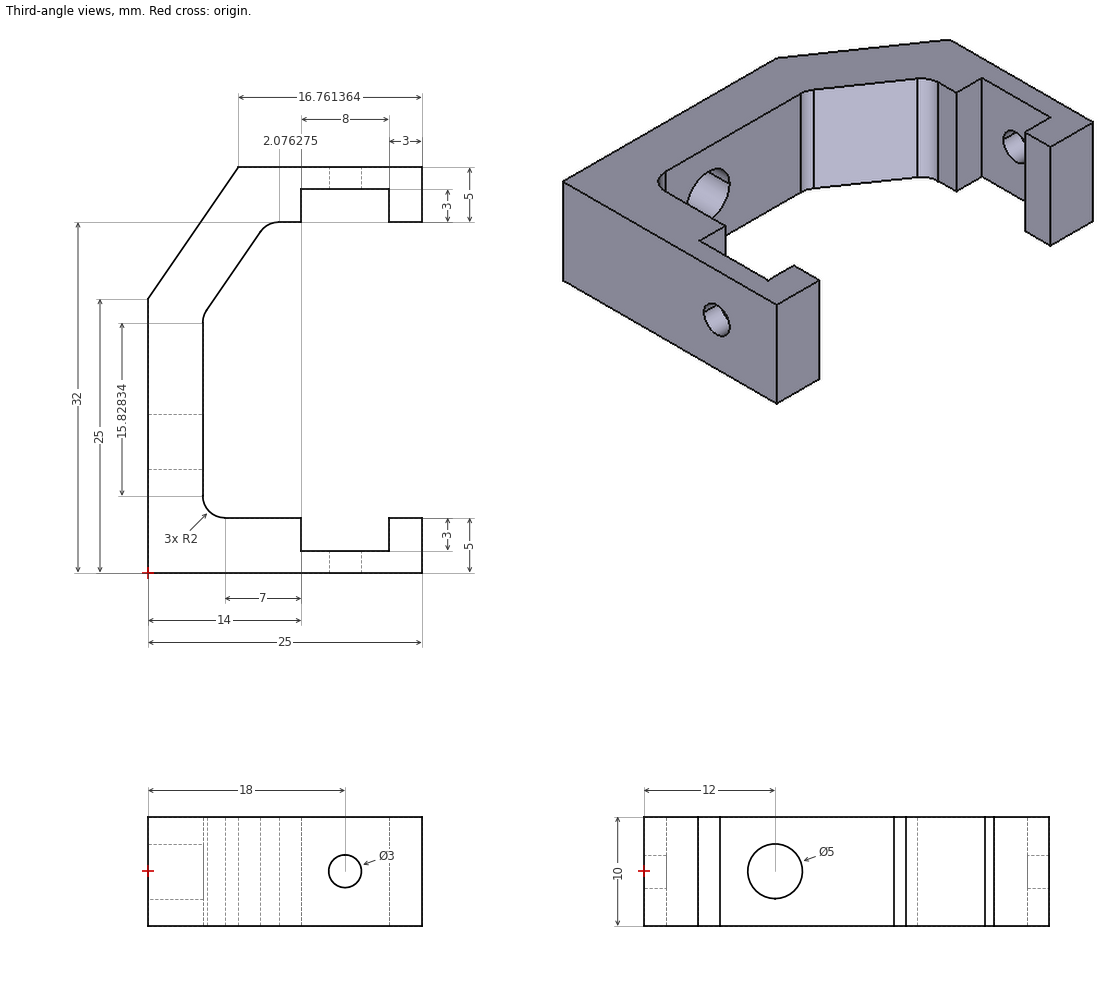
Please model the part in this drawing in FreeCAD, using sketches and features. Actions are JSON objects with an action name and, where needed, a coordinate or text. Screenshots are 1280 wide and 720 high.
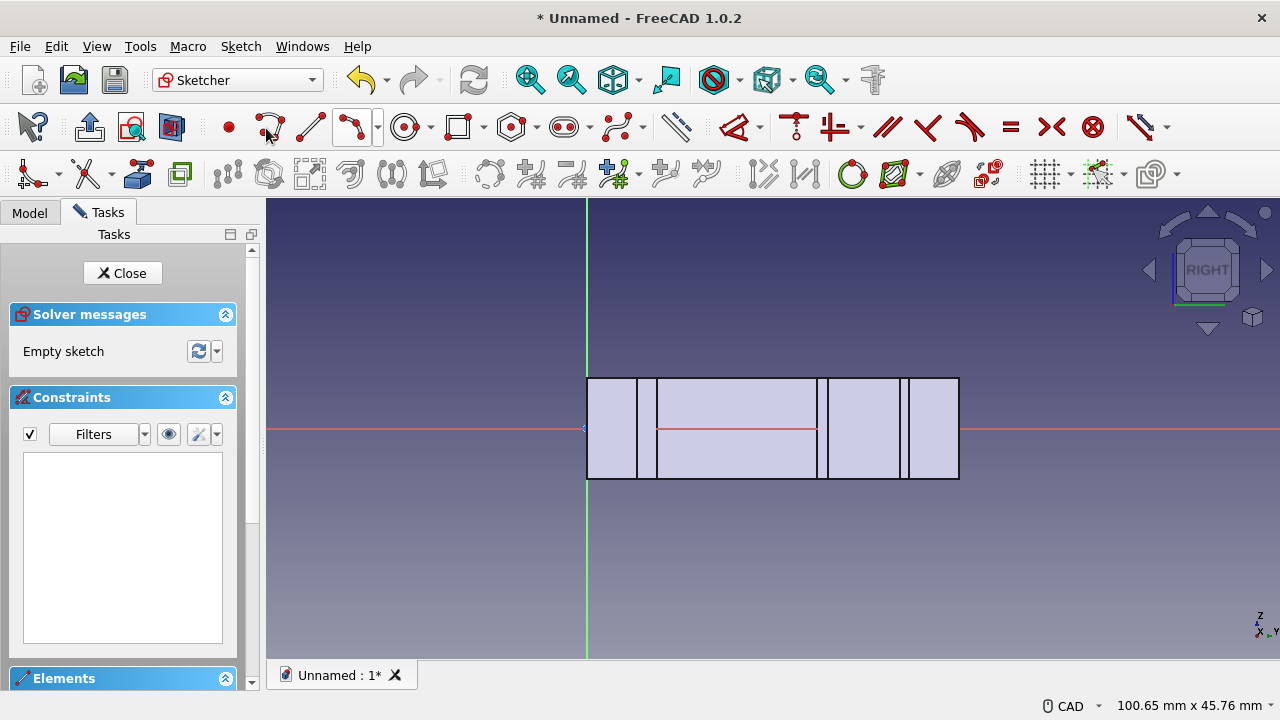
{"action": "scroll", "coordinate": [708, 428], "scroll_direction": "up", "scroll_amount": 9}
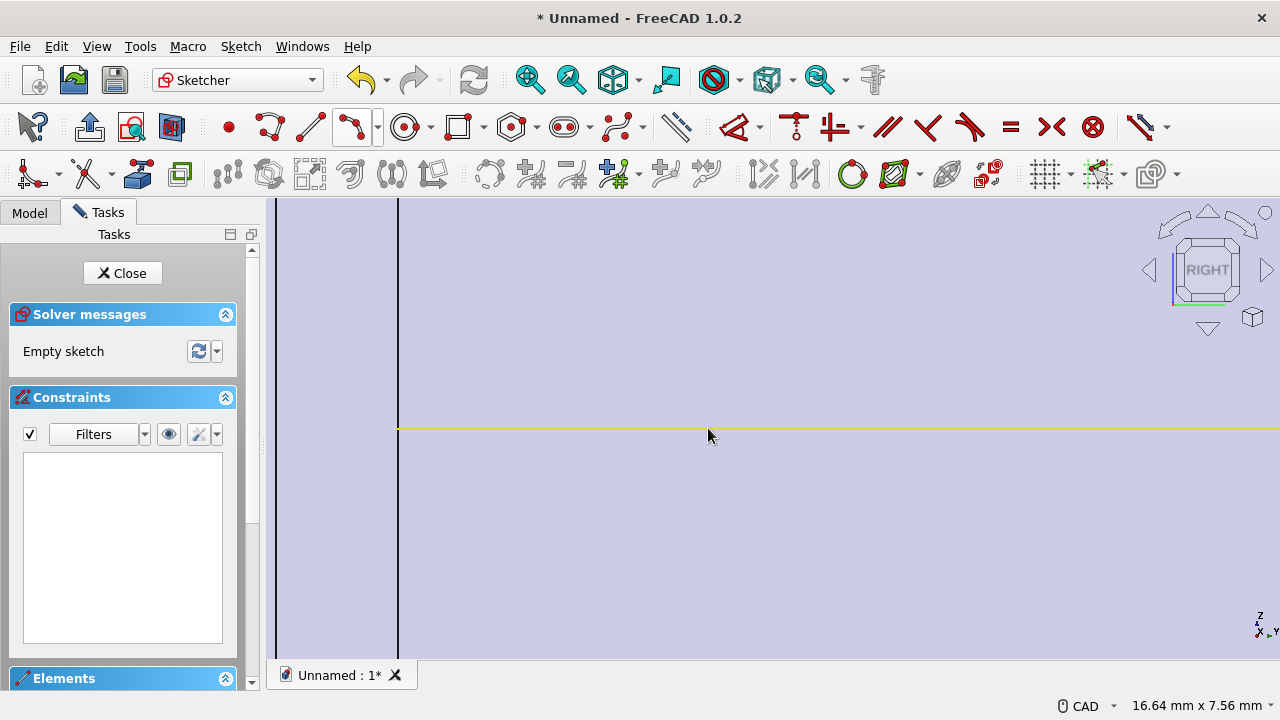
{"action": "left_click", "coordinate": [404, 128]}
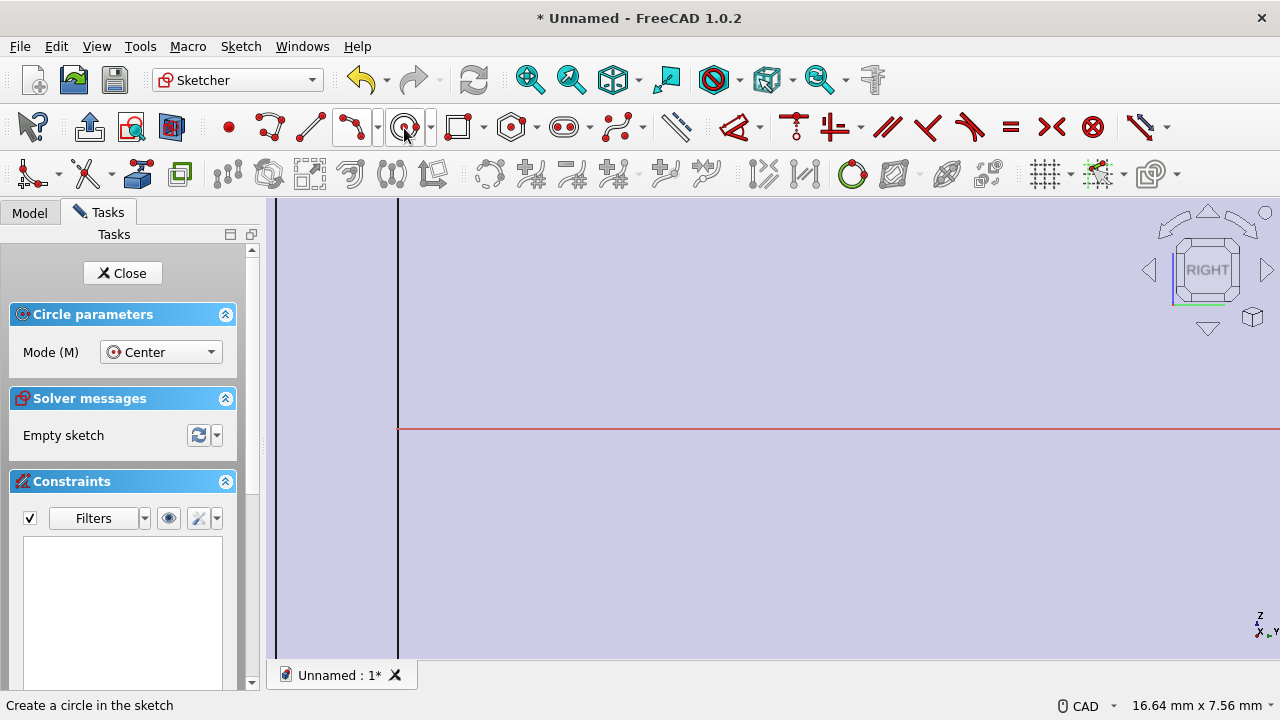
{"action": "left_click", "coordinate": [703, 428]}
{"action": "mouse_move", "coordinate": [811, 321]}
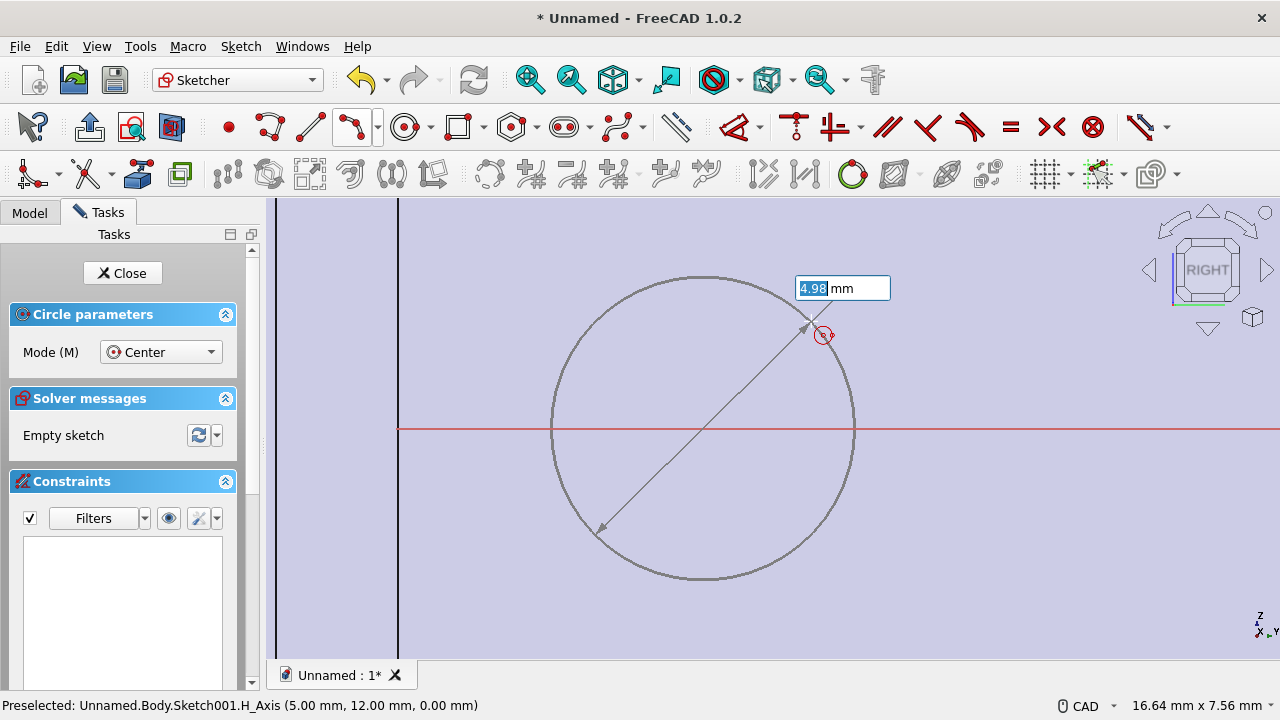
{"action": "type", "text": "5"}
{"action": "key", "text": "Return"}
{"action": "key", "text": "Escape"}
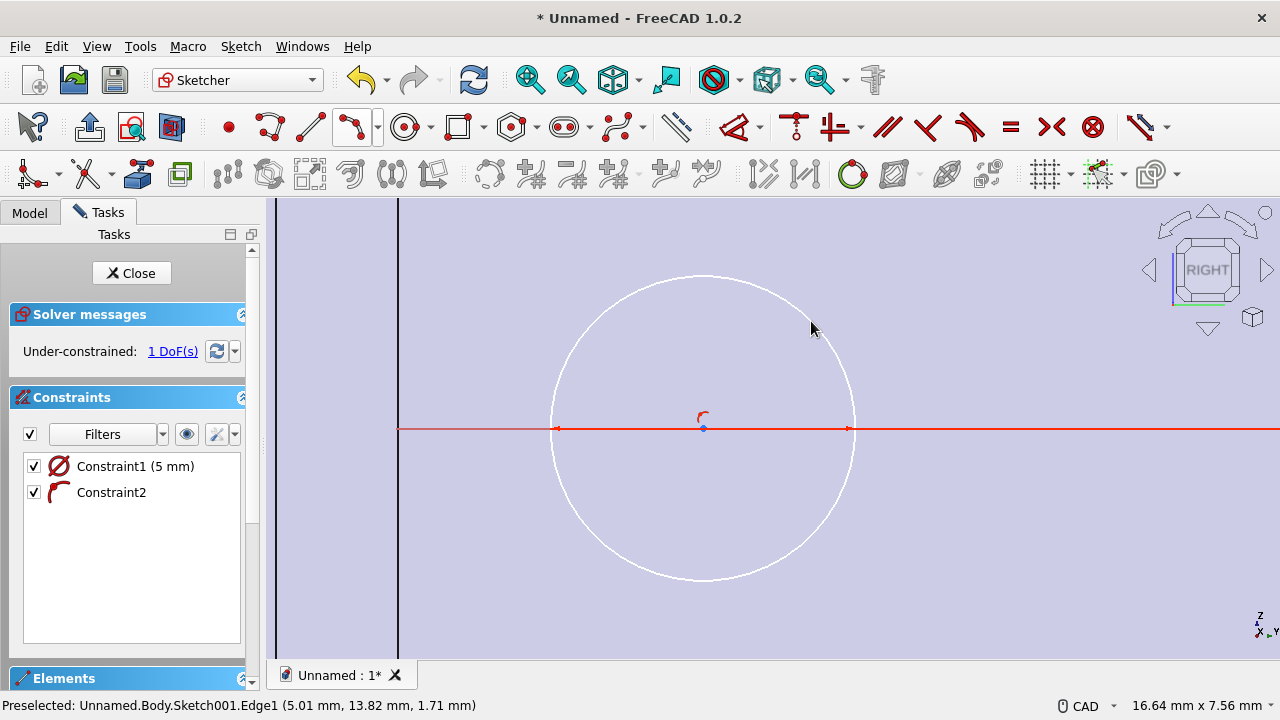
{"action": "left_click", "coordinate": [734, 128]}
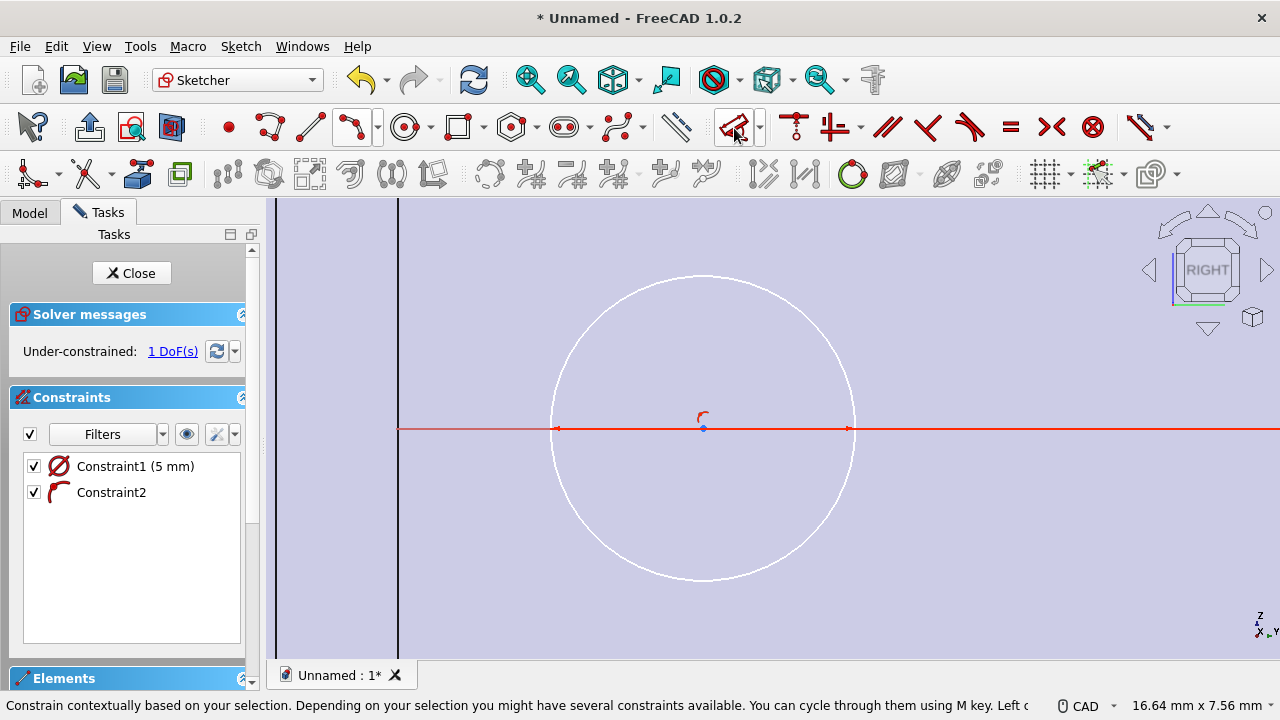
{"action": "left_click", "coordinate": [703, 428]}
{"action": "left_click", "coordinate": [499, 462]}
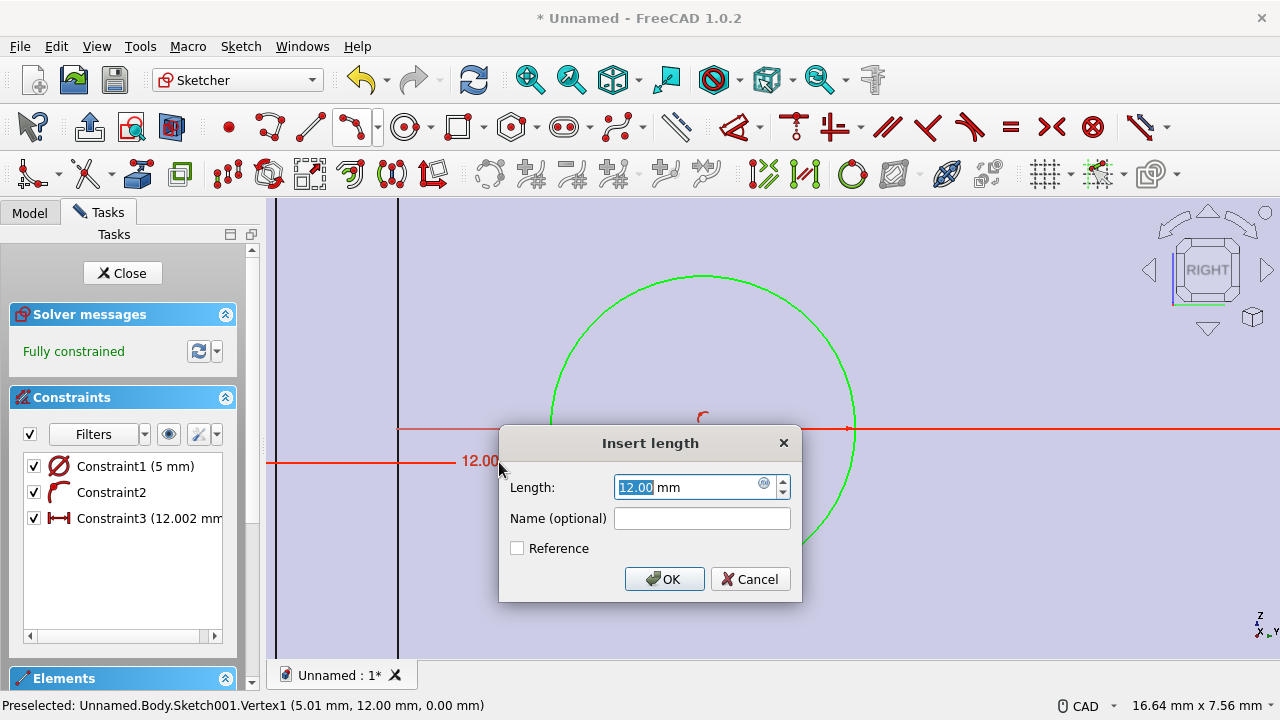
{"action": "type", "text": "12"}
{"action": "key", "text": "Return"}
{"action": "key", "text": "Escape"}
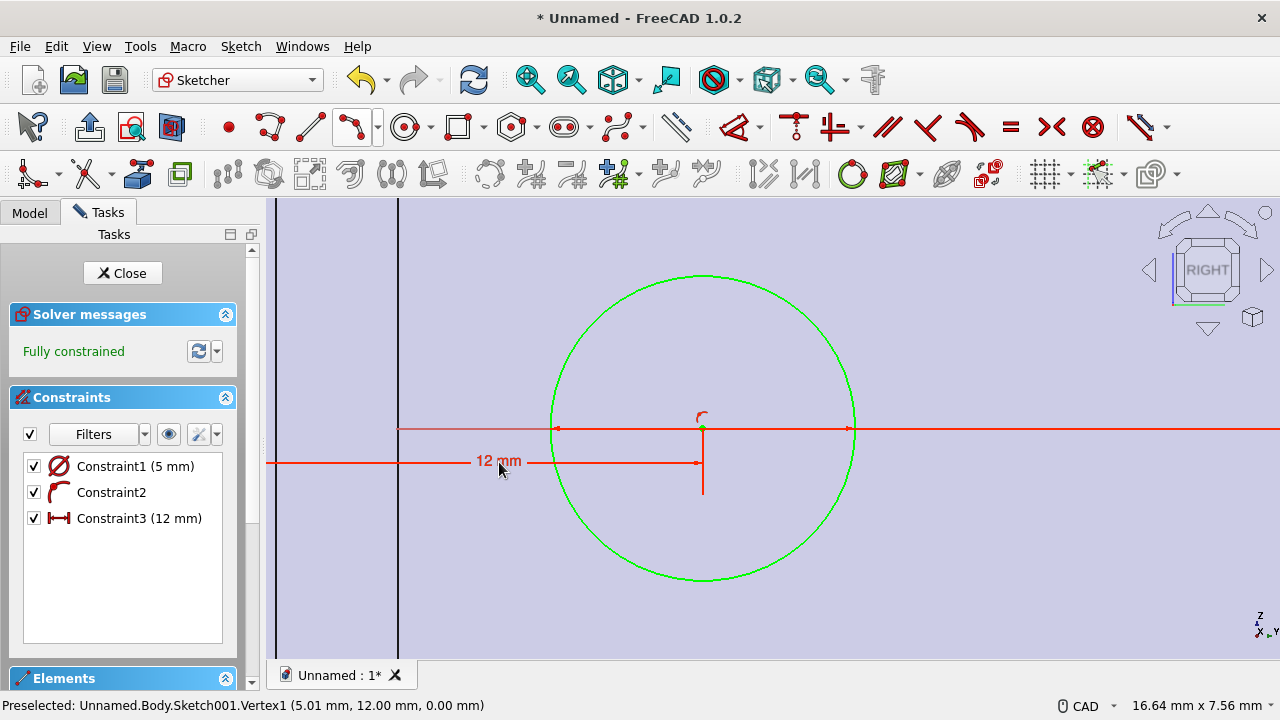
{"action": "left_click", "coordinate": [123, 273]}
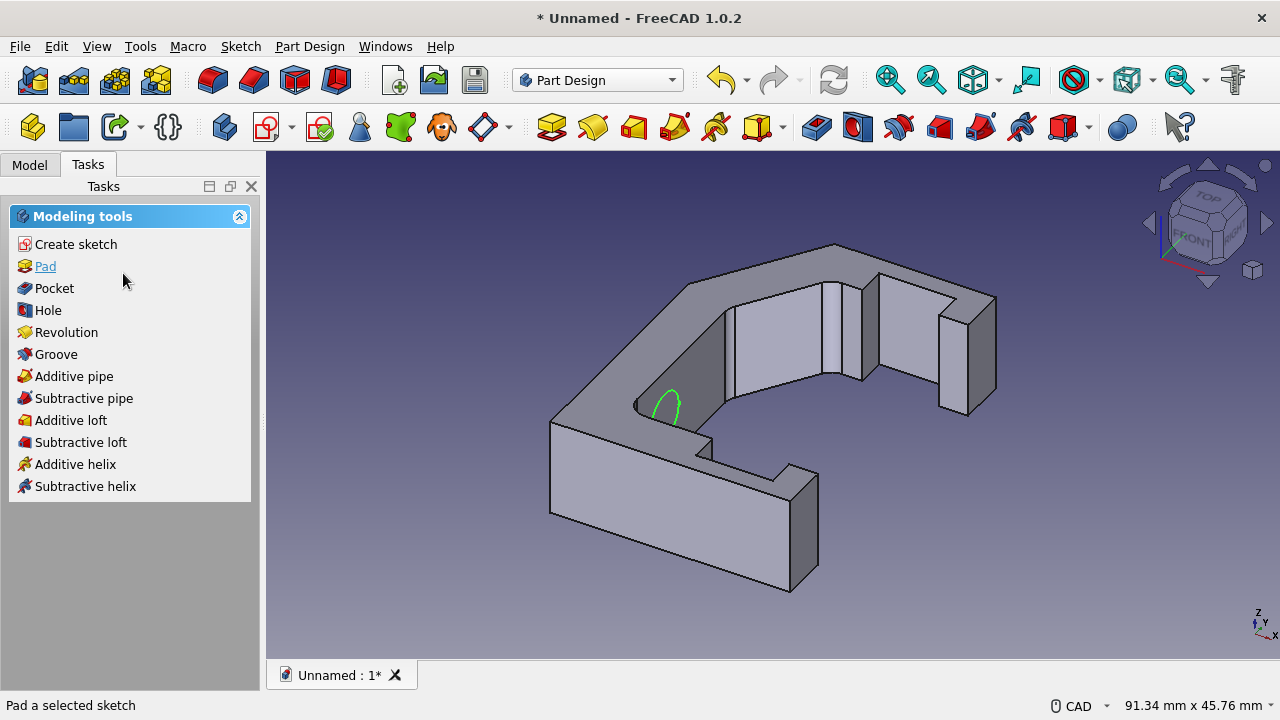
{"action": "left_click", "coordinate": [817, 128]}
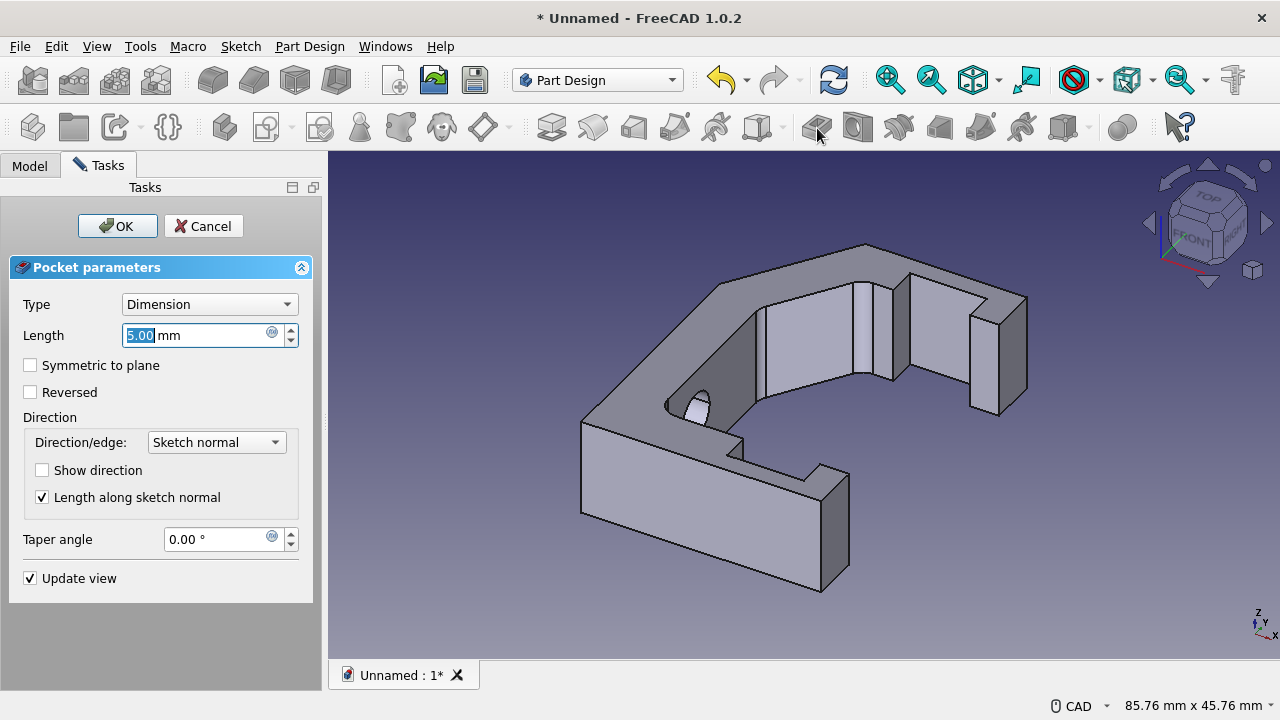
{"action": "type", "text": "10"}
{"action": "key", "text": "Tab"}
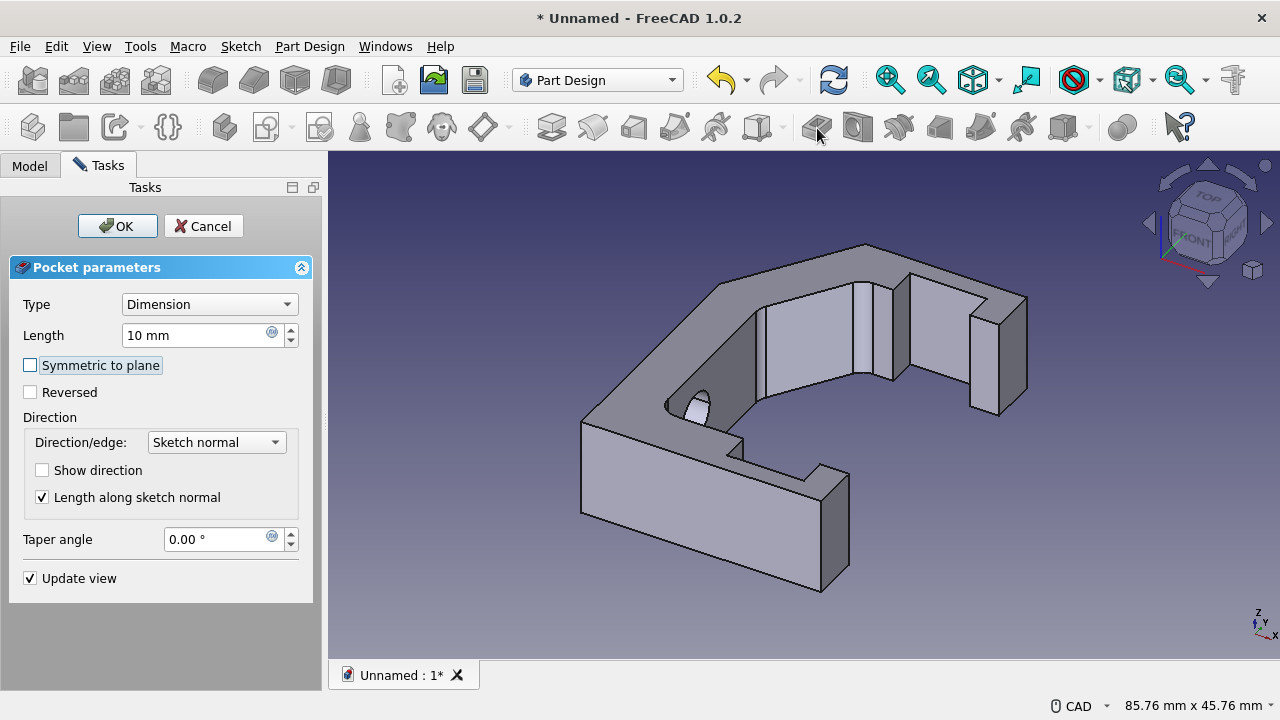
{"action": "left_click", "coordinate": [118, 226]}